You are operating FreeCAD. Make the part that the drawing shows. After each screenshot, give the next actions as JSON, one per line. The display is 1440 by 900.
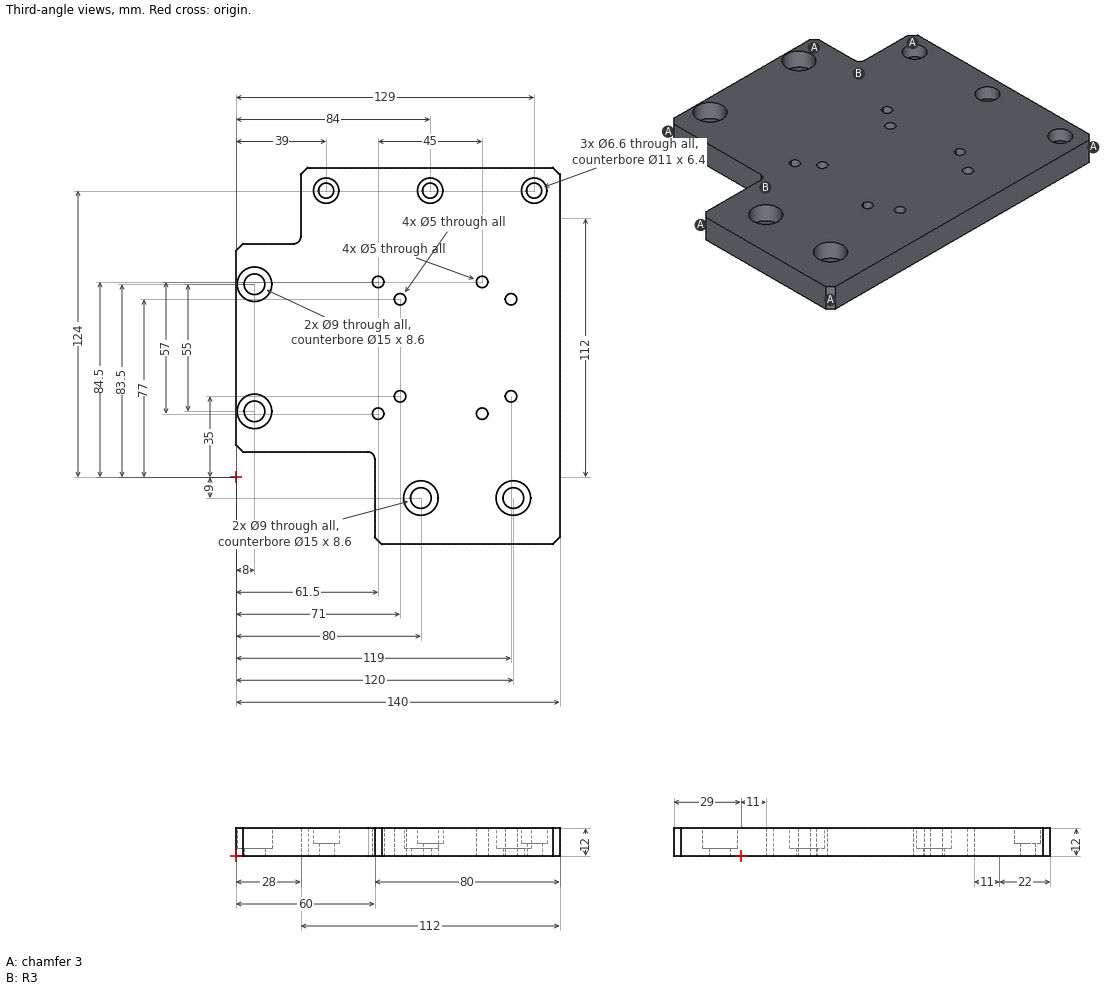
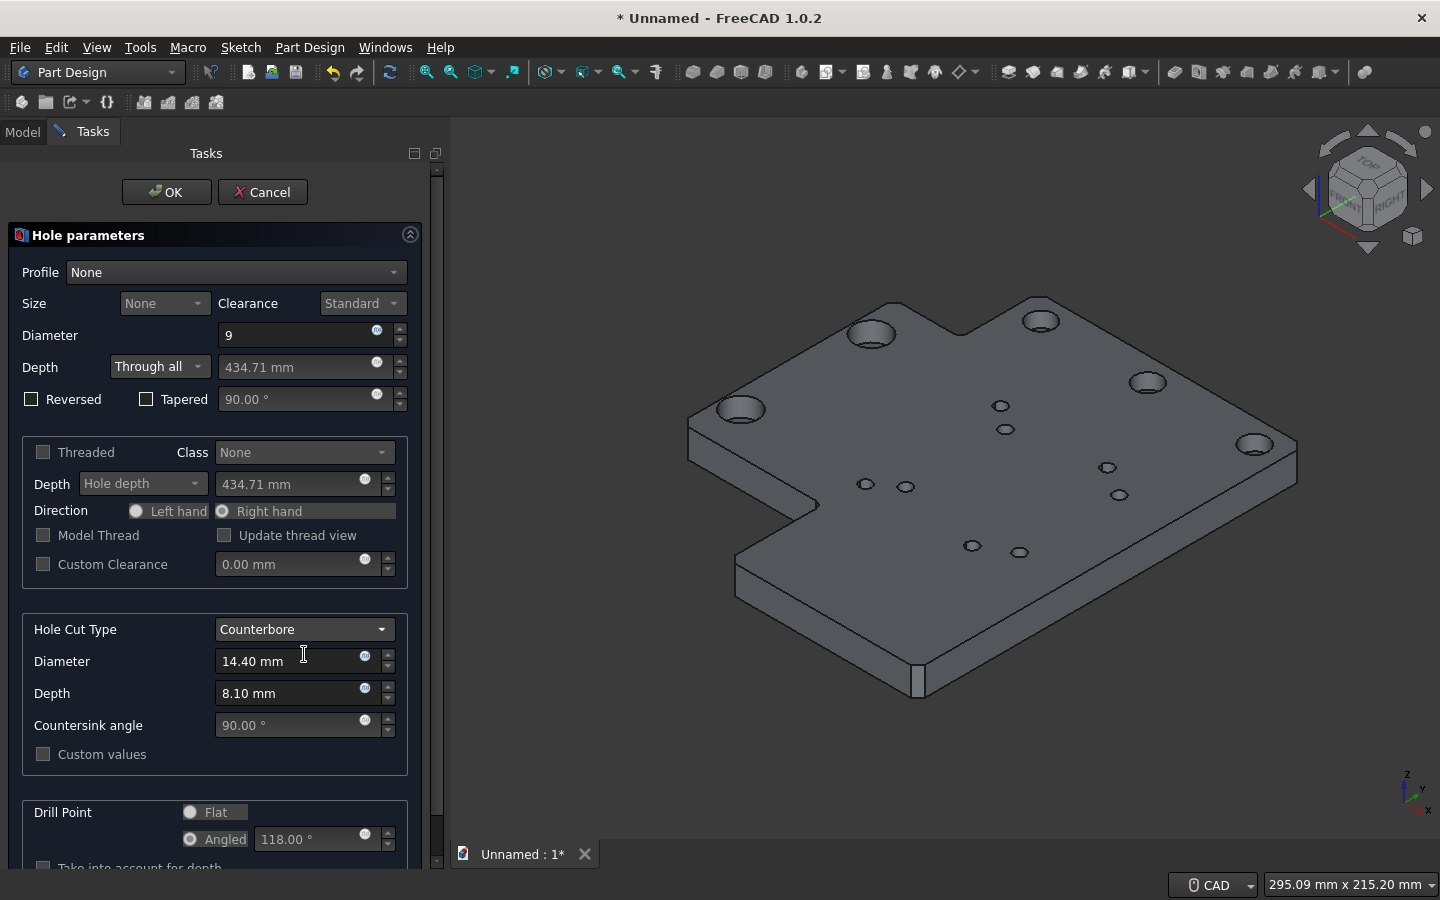
{"action": "triple_click", "coordinate": [298, 661]}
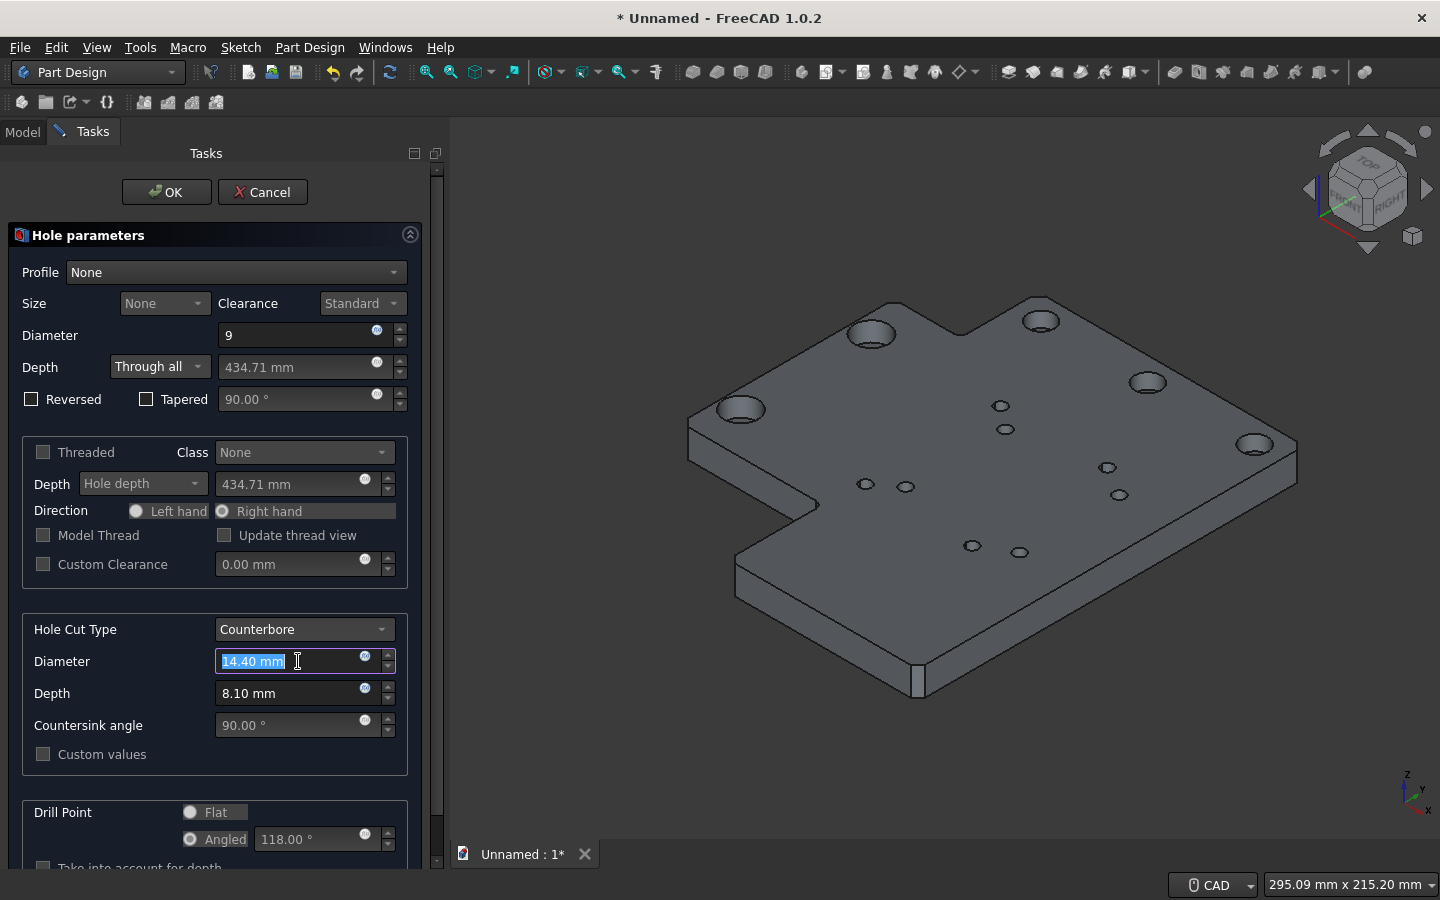
{"action": "type", "text": "15"}
{"action": "key", "text": "Tab"}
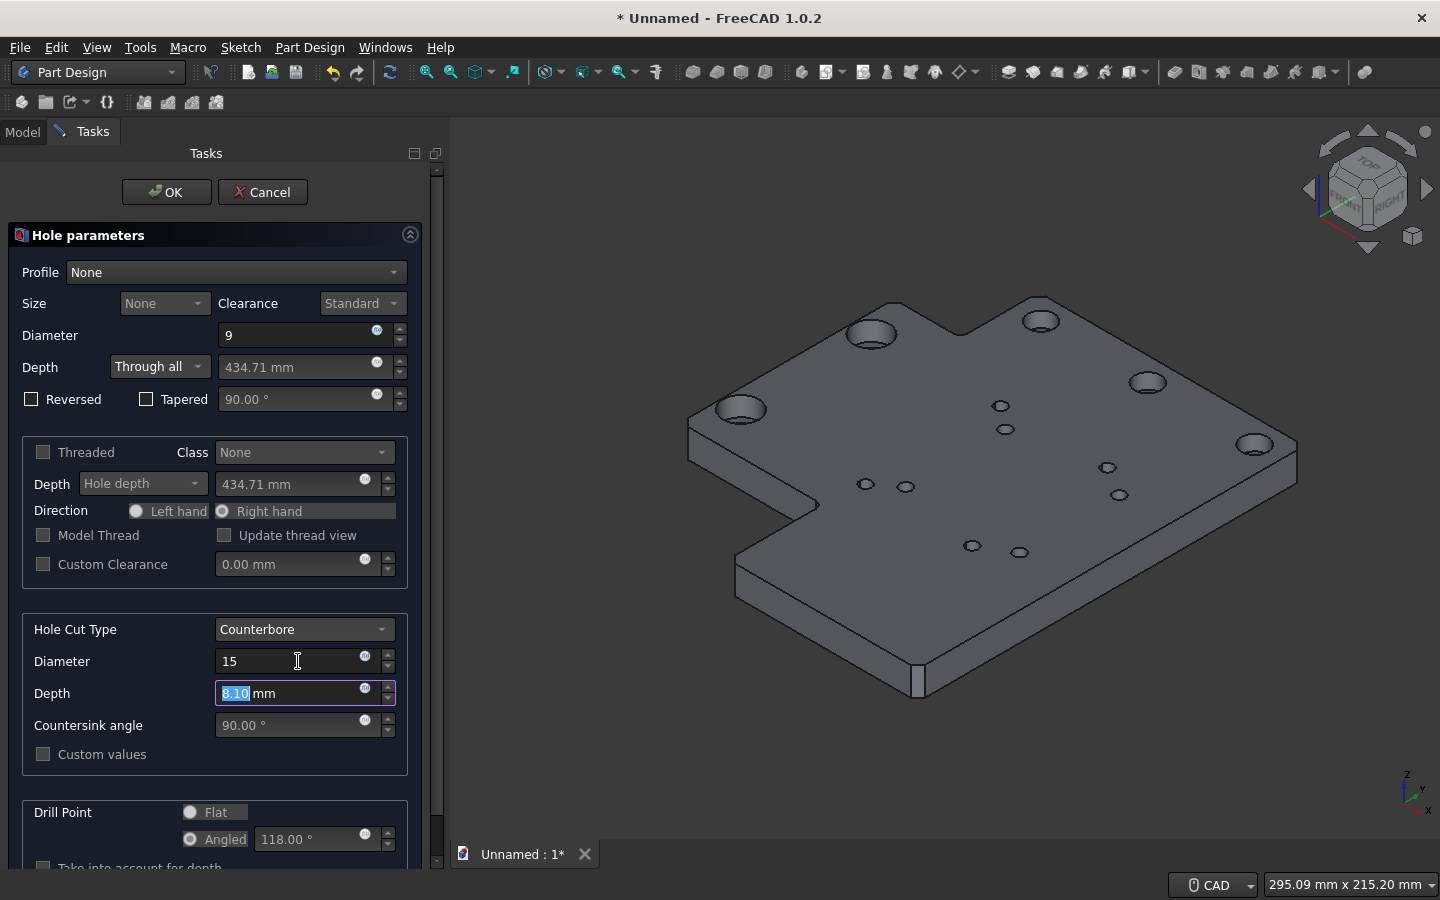
{"action": "type", "text": "8.6"}
{"action": "key", "text": "Tab"}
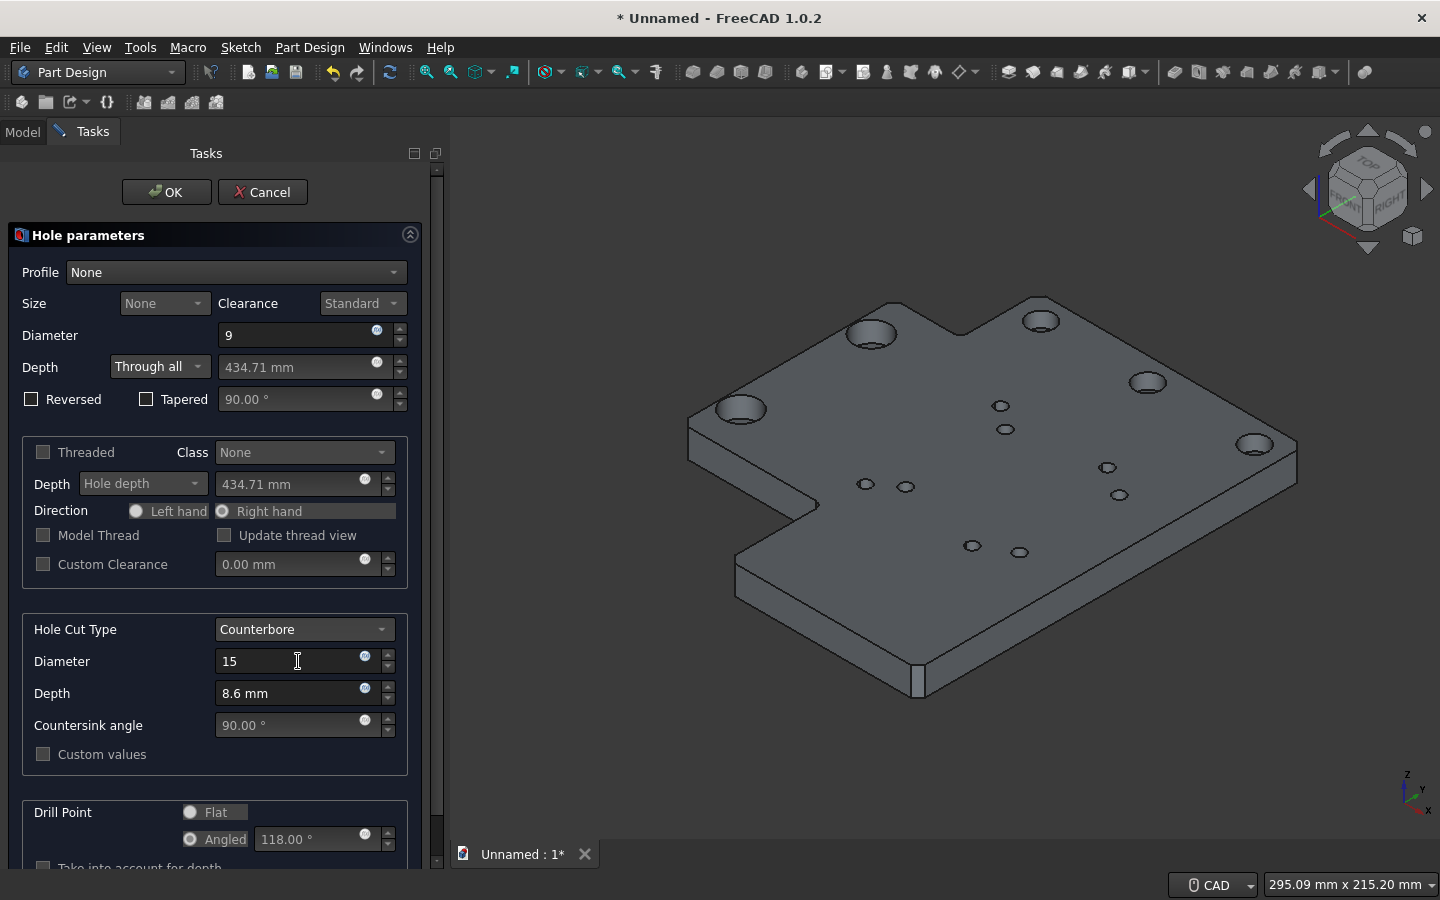
{"action": "left_click", "coordinate": [167, 192]}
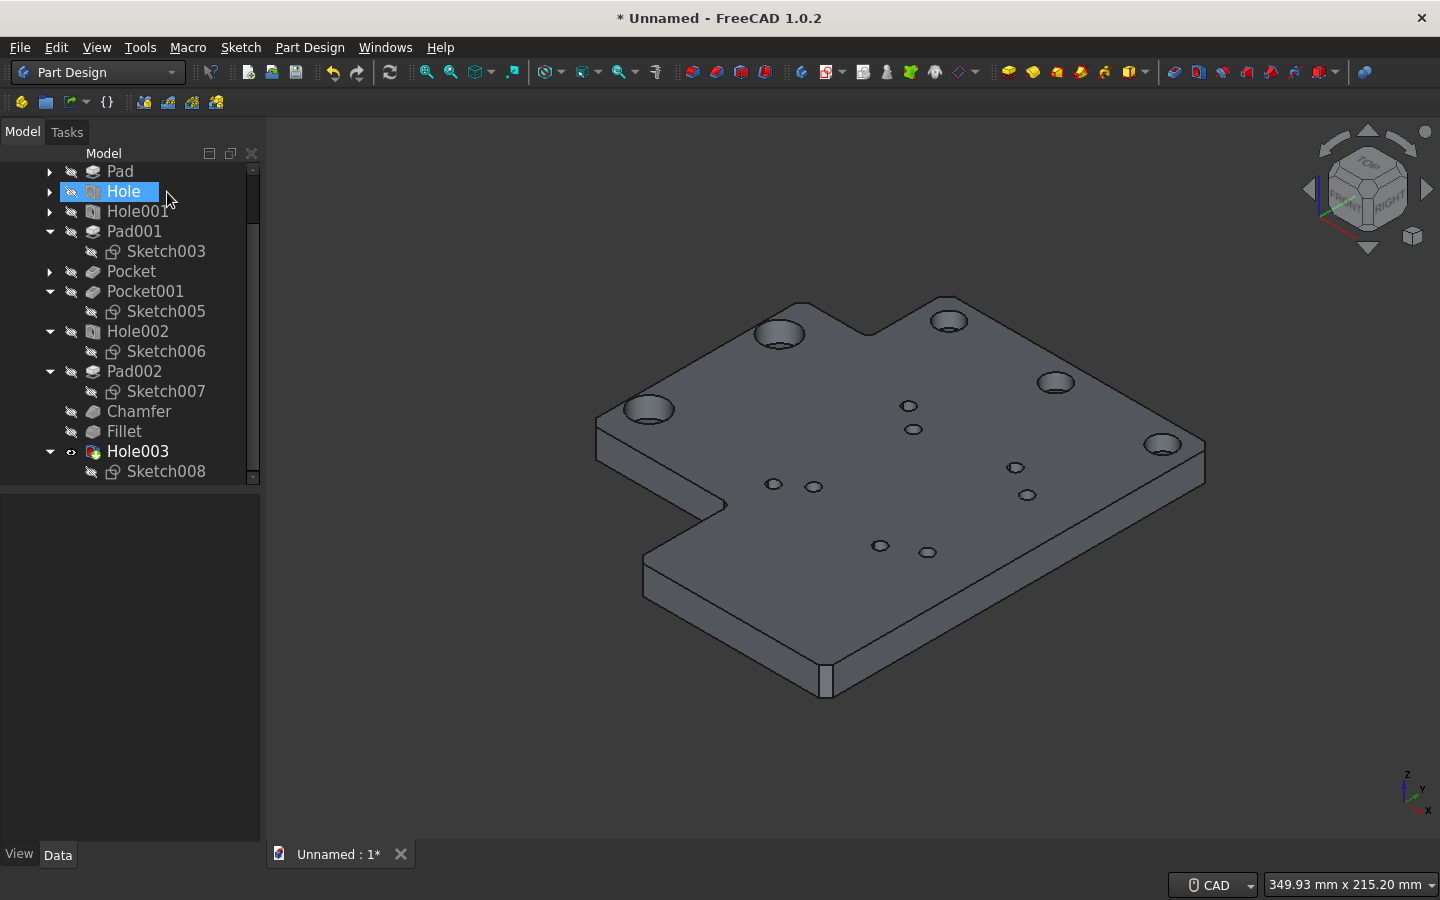
{"action": "left_click", "coordinate": [758, 406]}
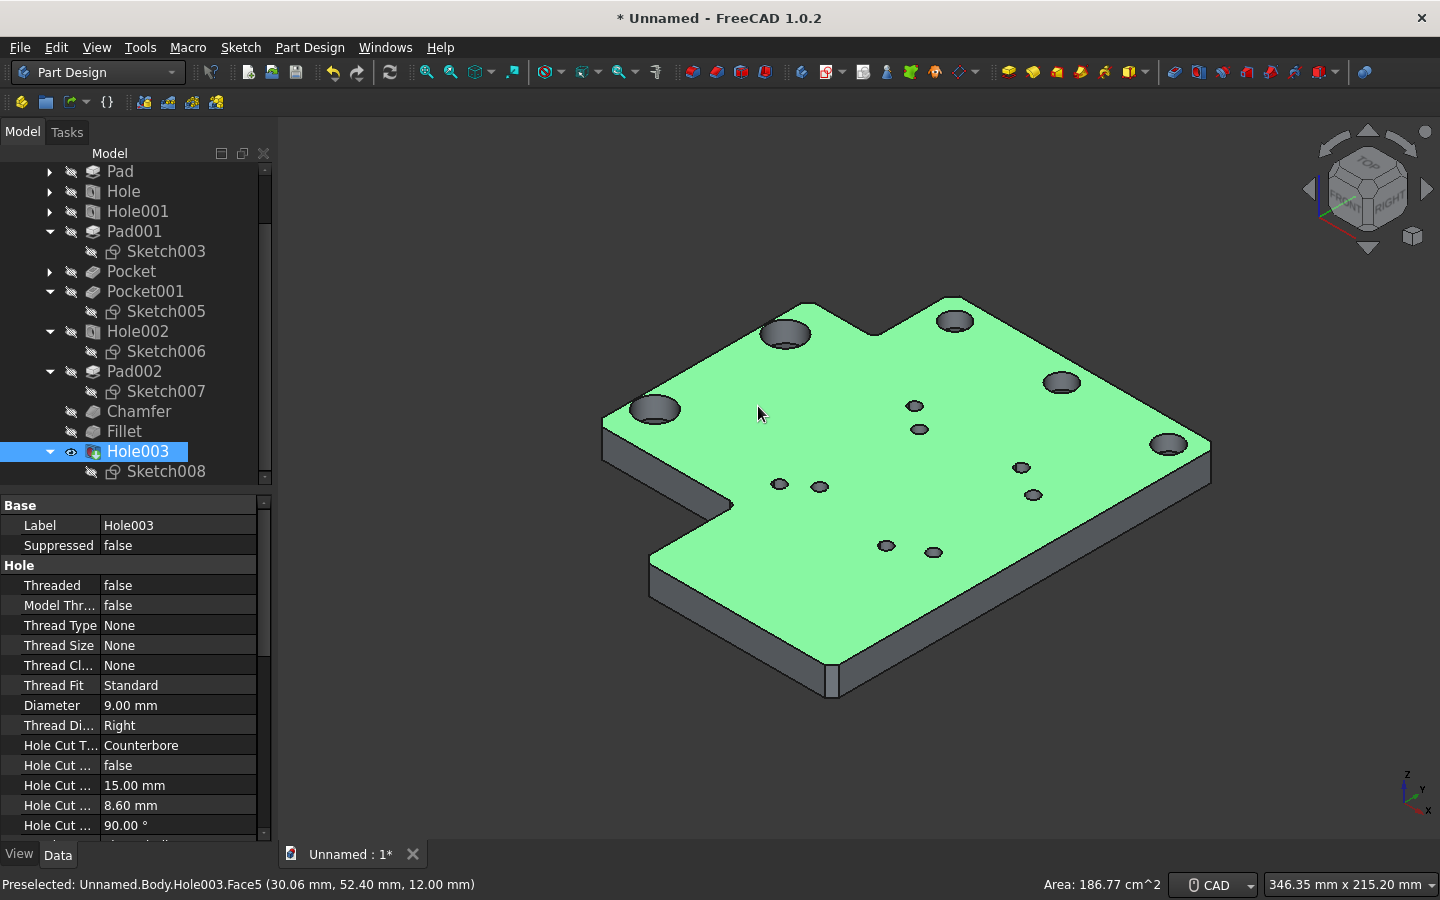
{"action": "left_click", "coordinate": [826, 72]}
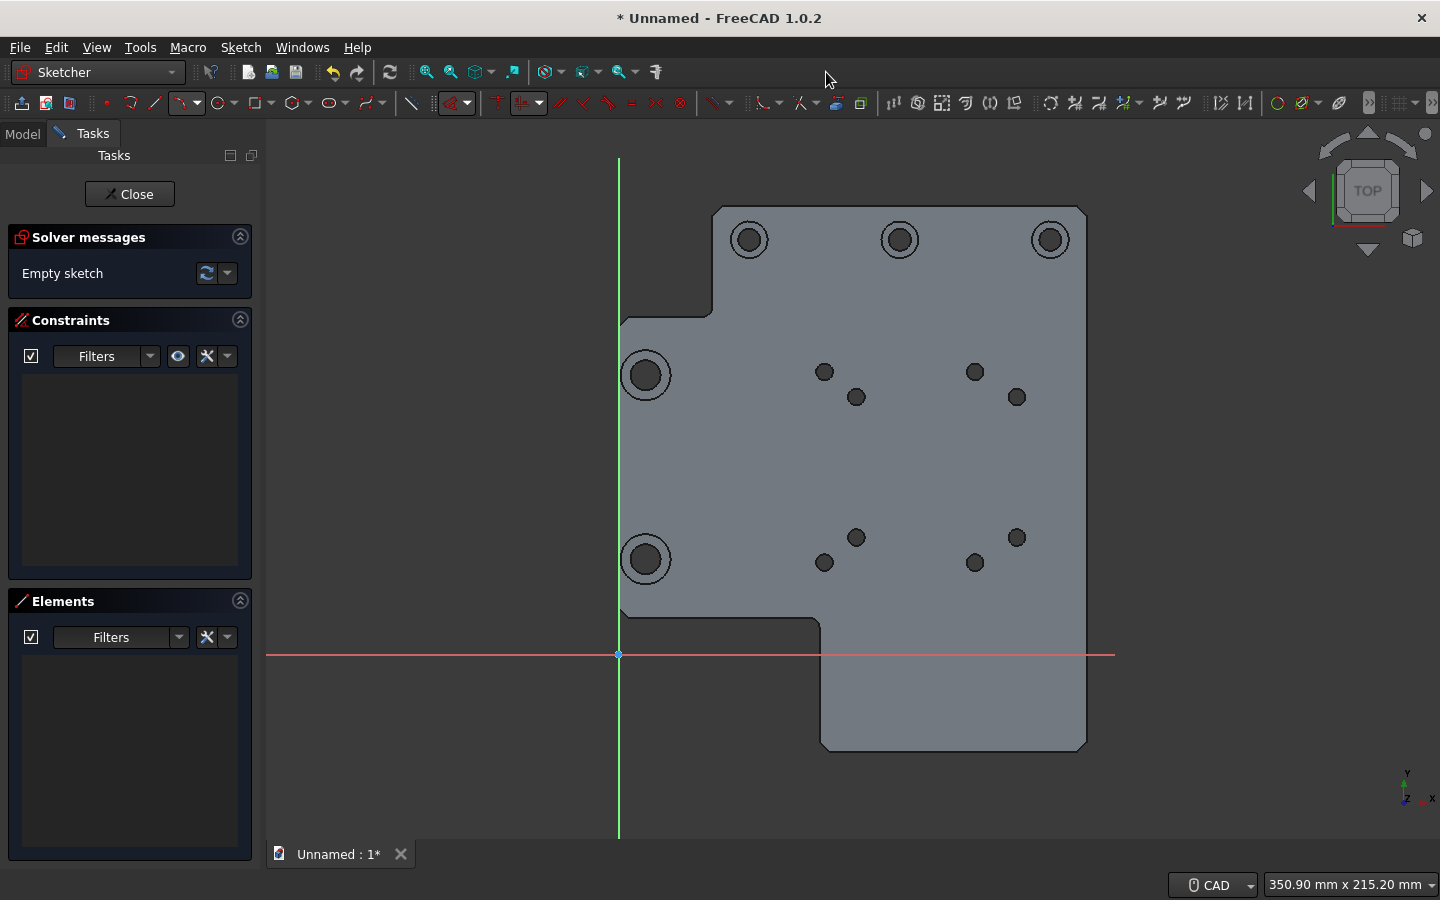
{"action": "scroll", "coordinate": [1009, 752], "scroll_direction": "up", "scroll_amount": 7}